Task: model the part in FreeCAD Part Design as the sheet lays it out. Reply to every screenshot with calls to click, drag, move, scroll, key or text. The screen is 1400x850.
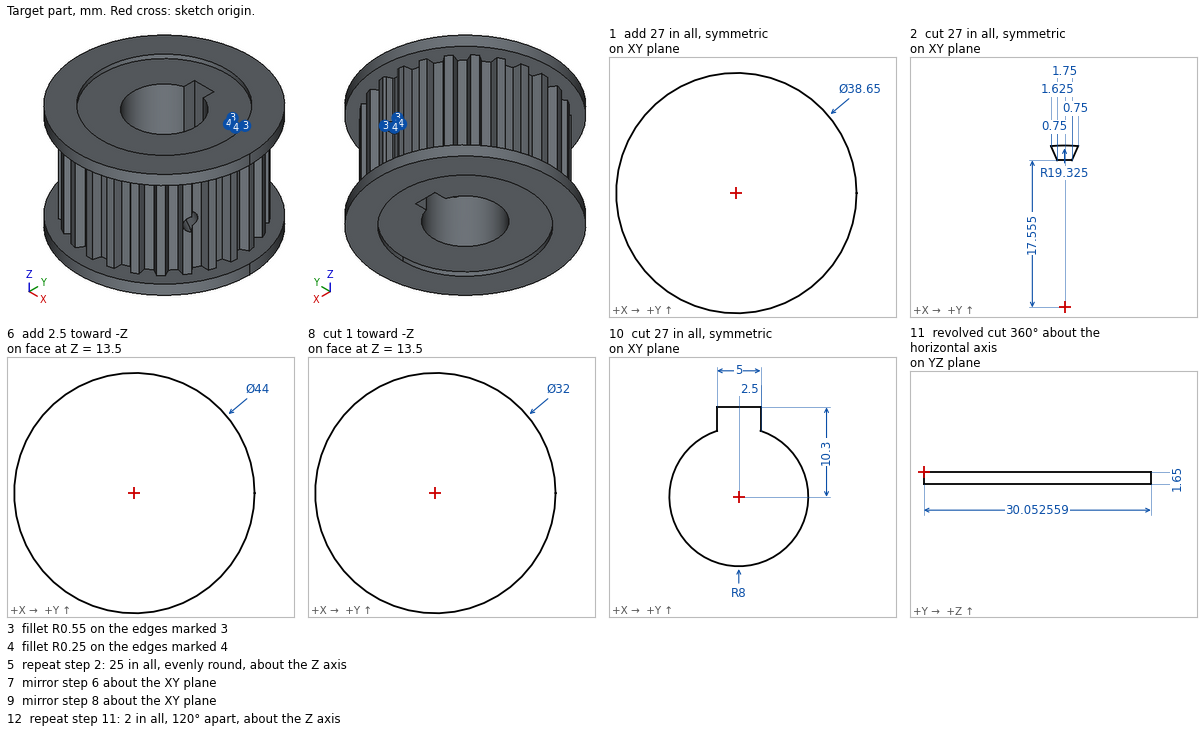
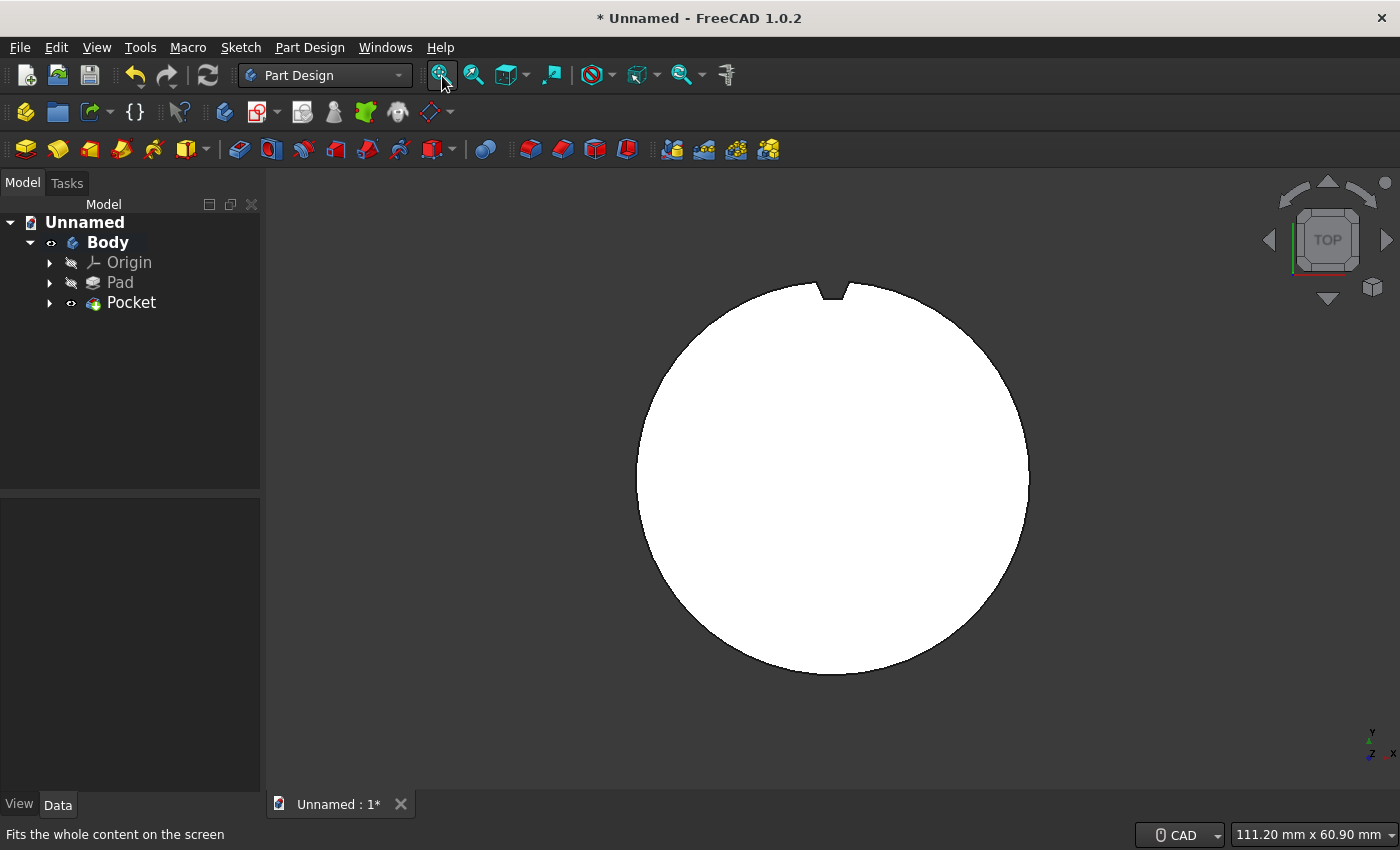
key(1)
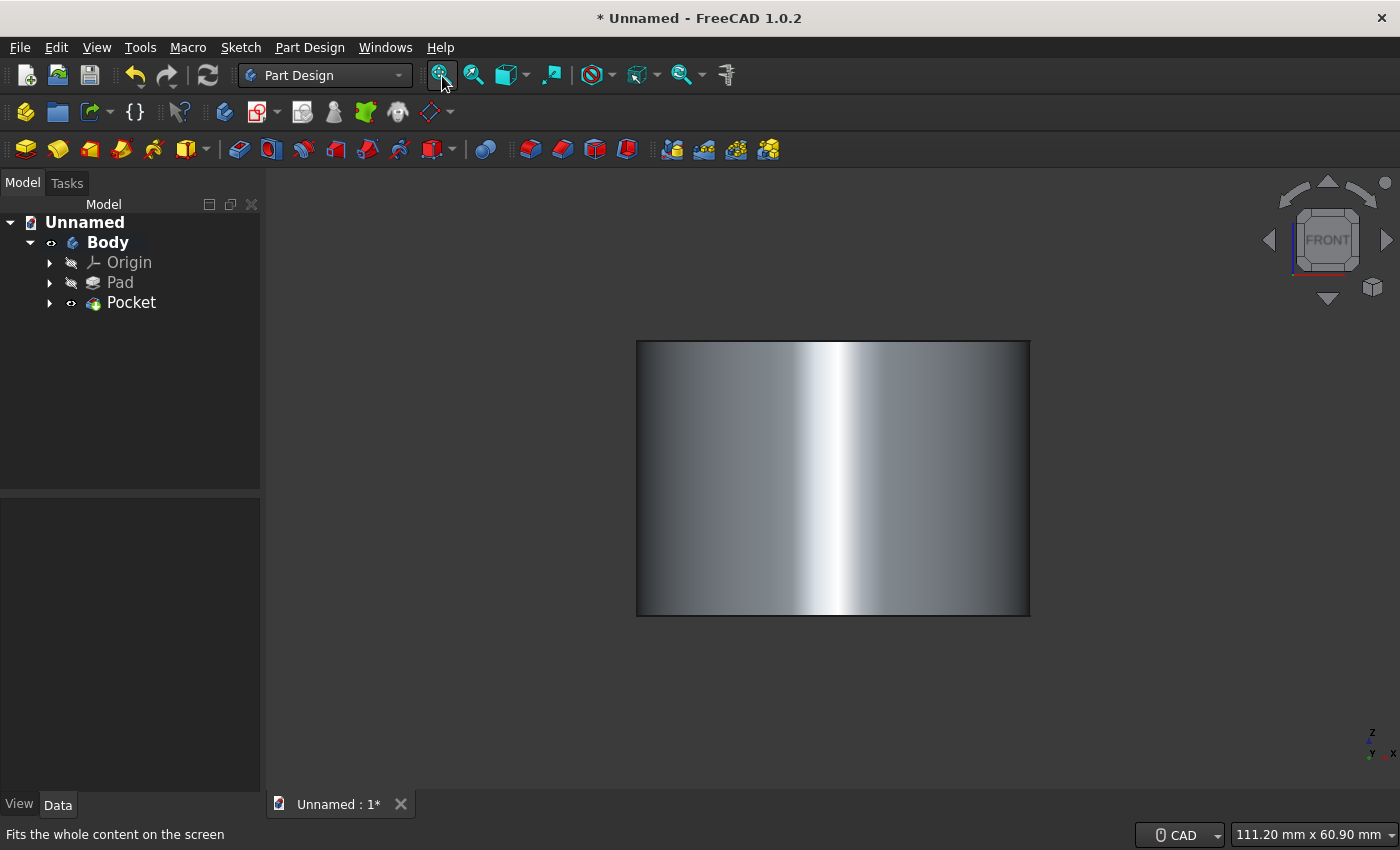
click(442, 76)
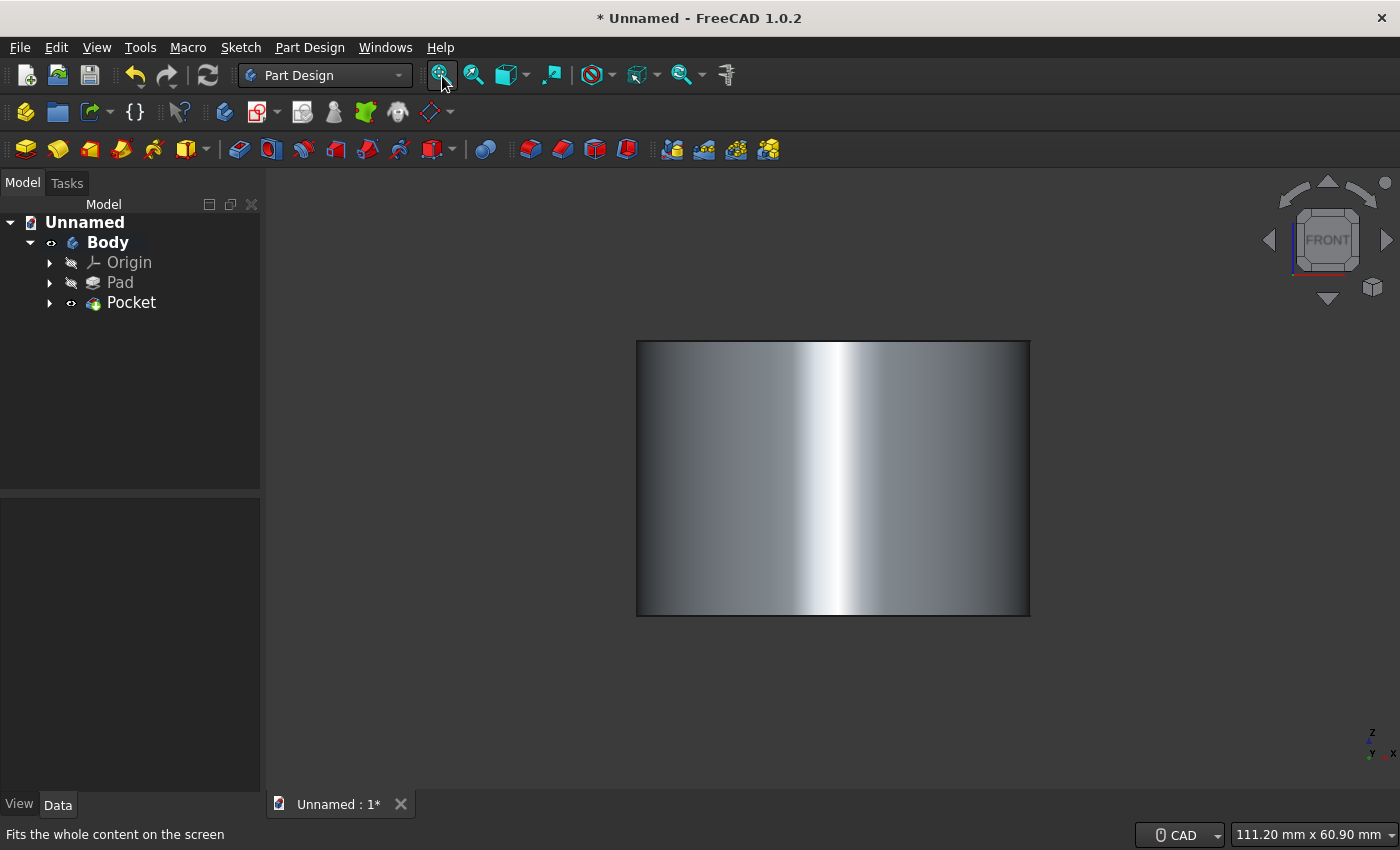
key(3)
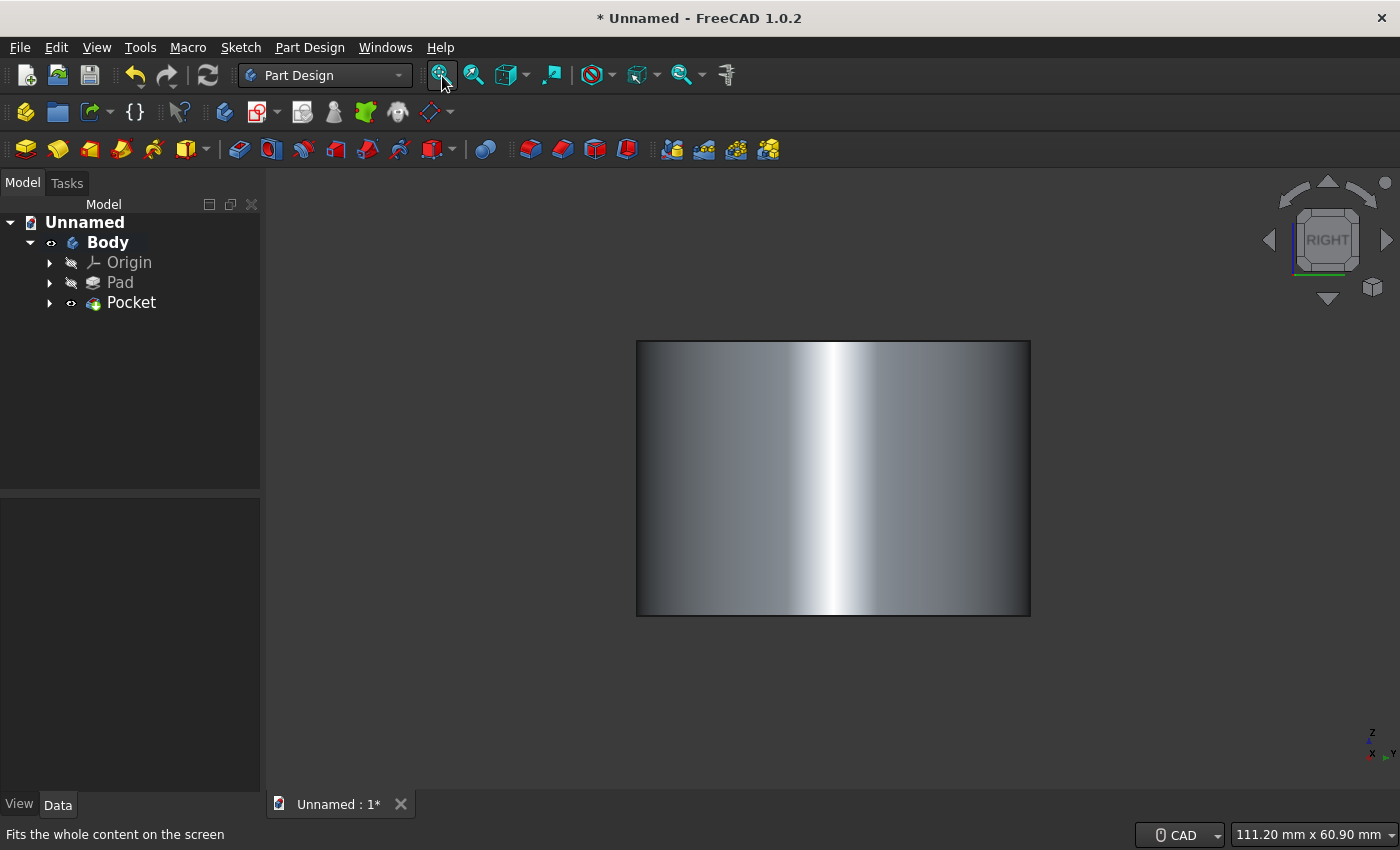
click(442, 76)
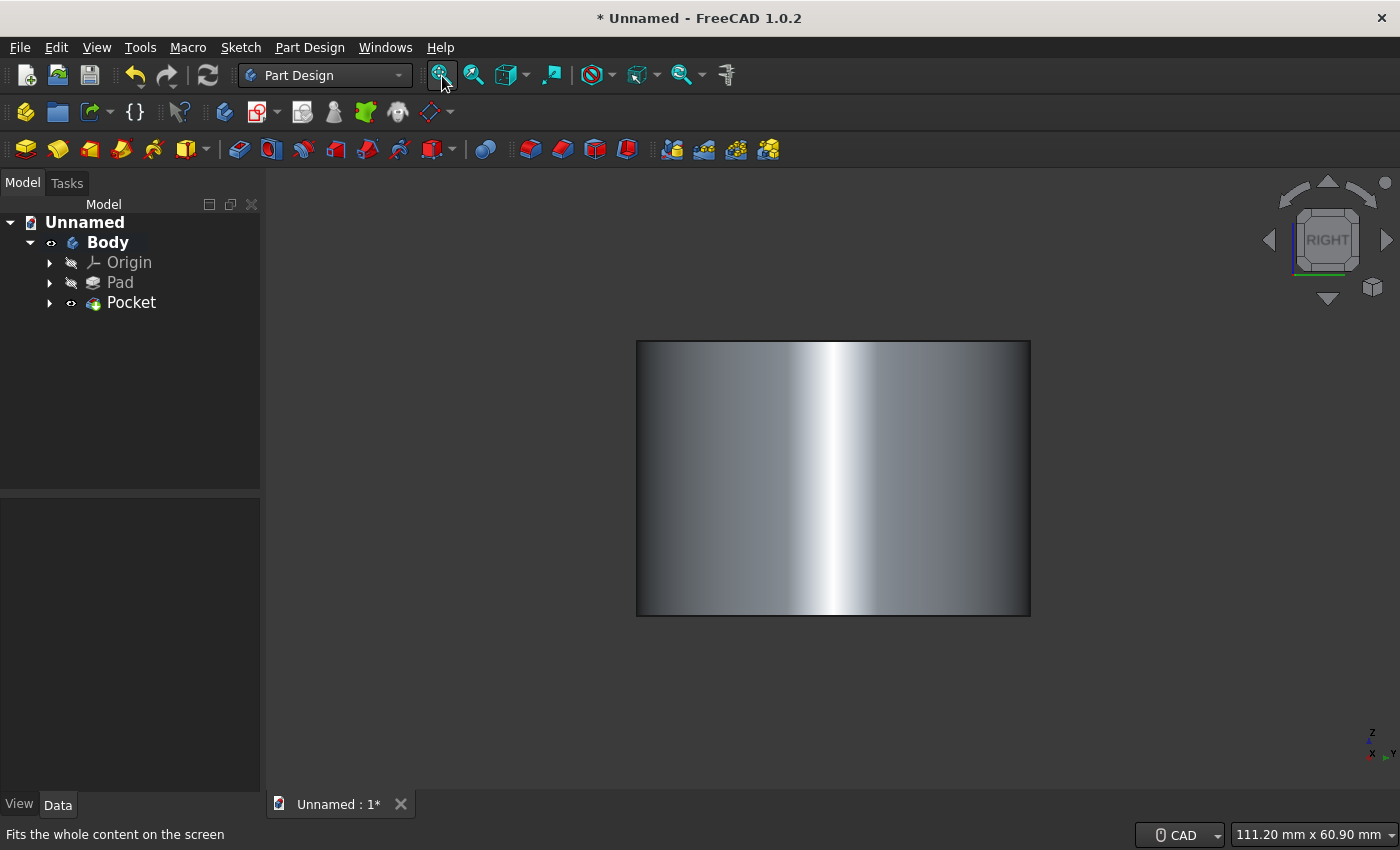
key(5)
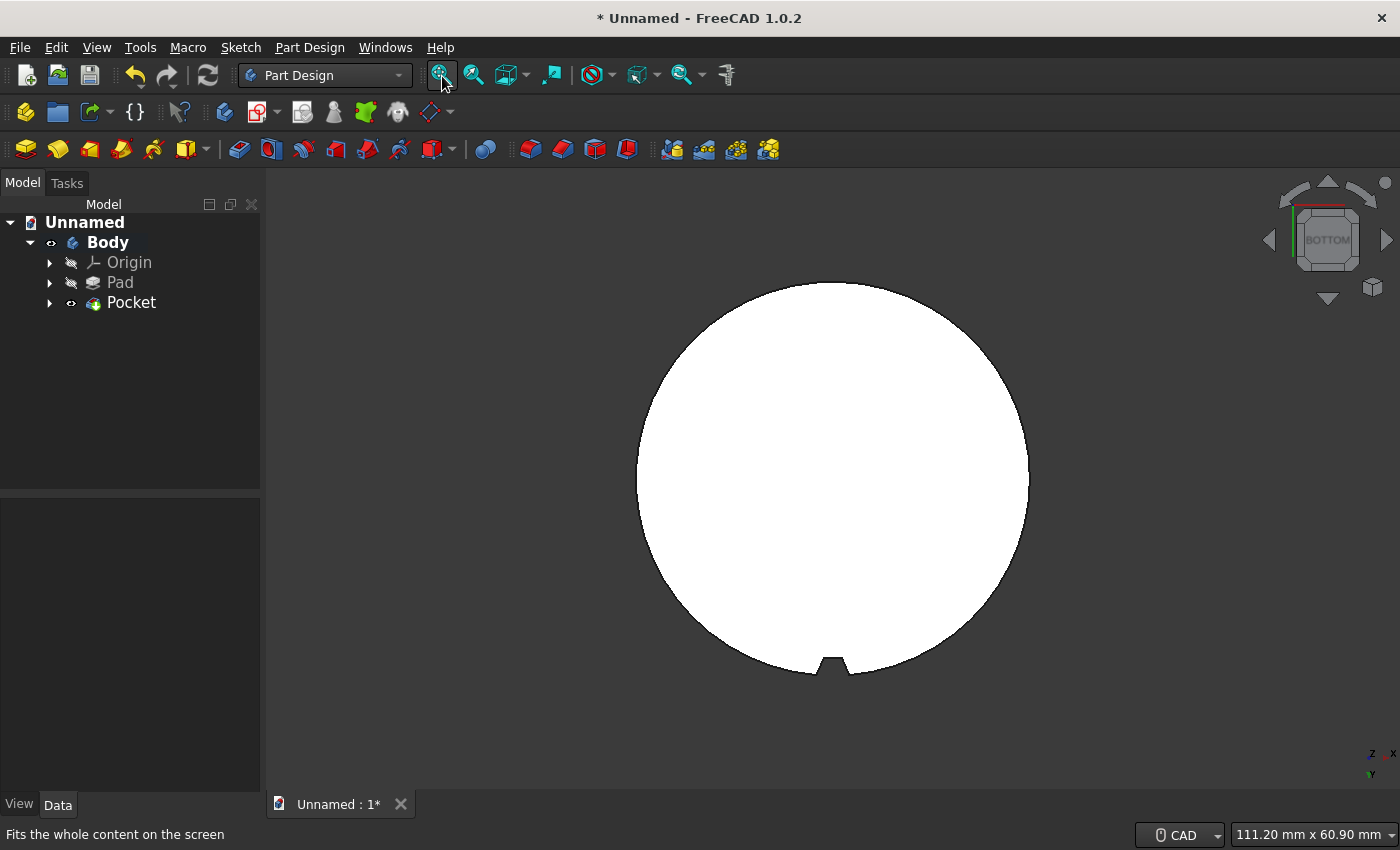
key(4)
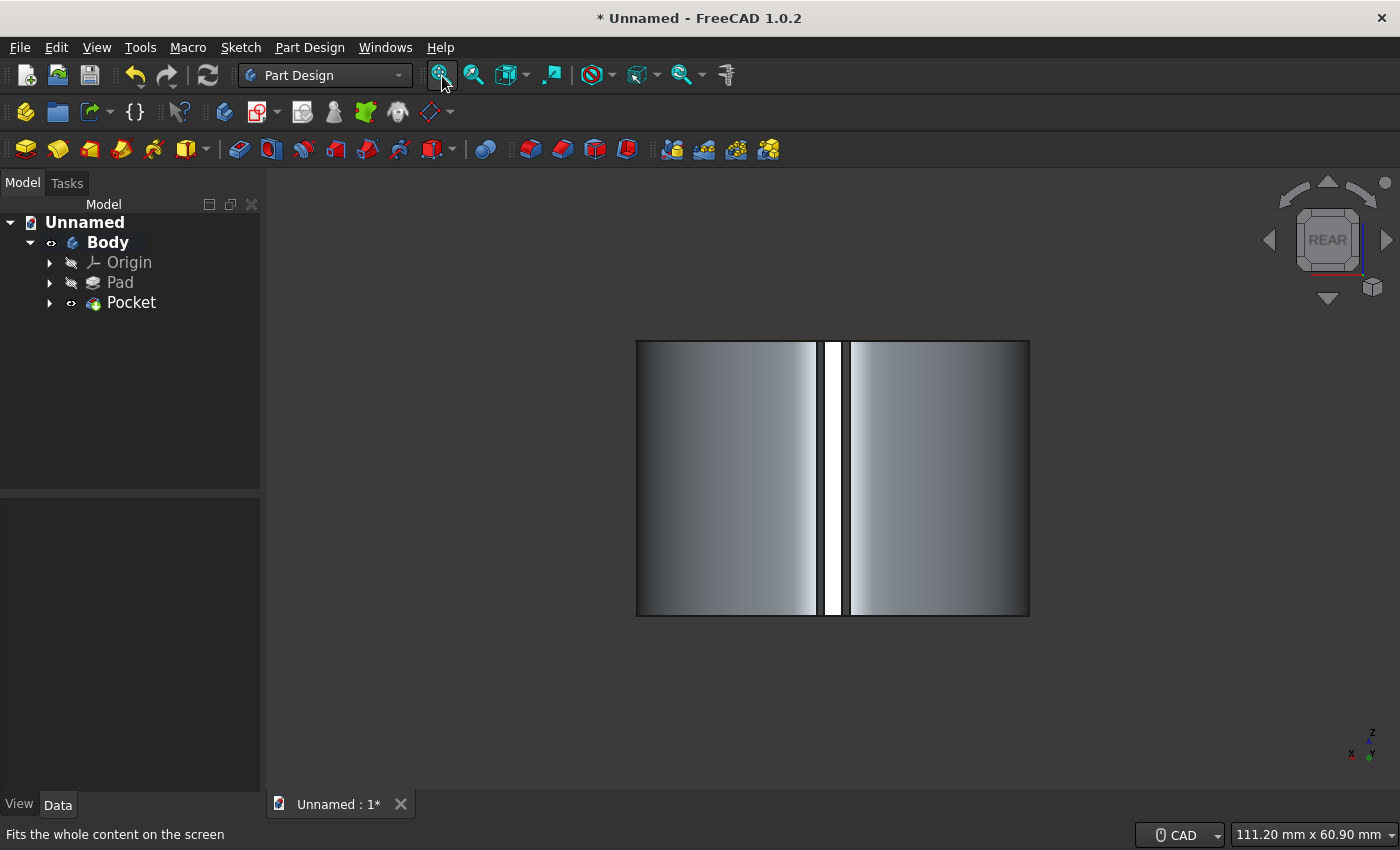
click(442, 76)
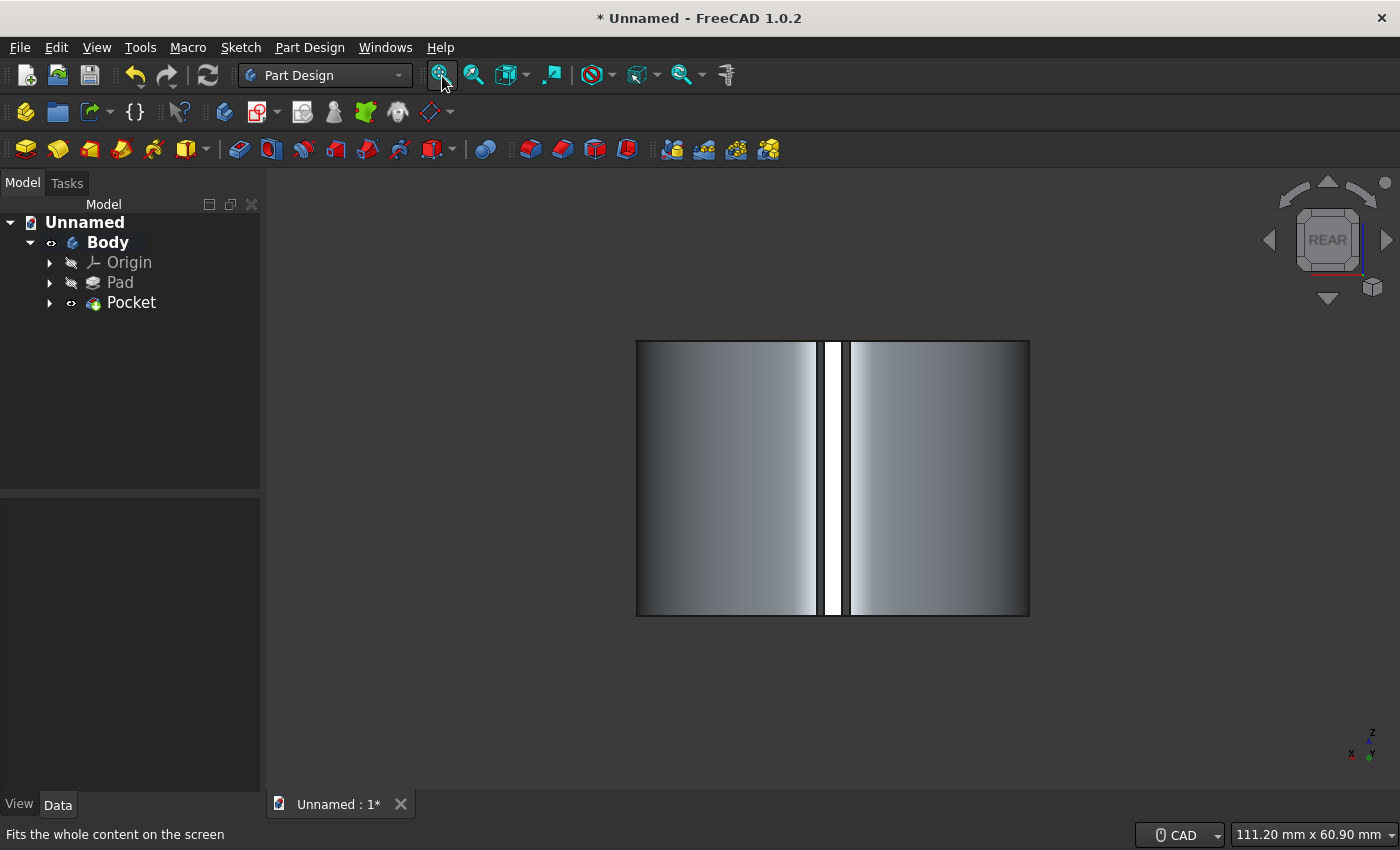
click(850, 478)